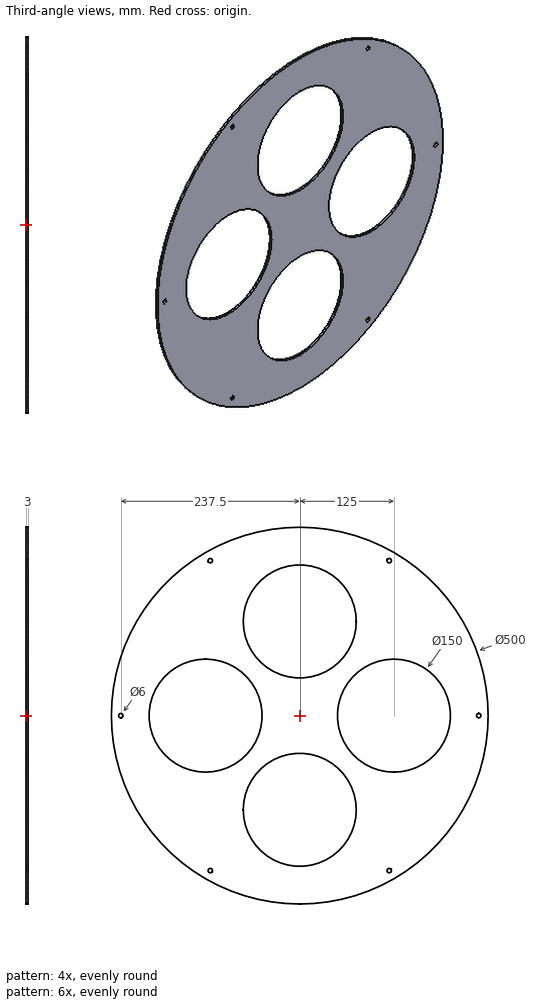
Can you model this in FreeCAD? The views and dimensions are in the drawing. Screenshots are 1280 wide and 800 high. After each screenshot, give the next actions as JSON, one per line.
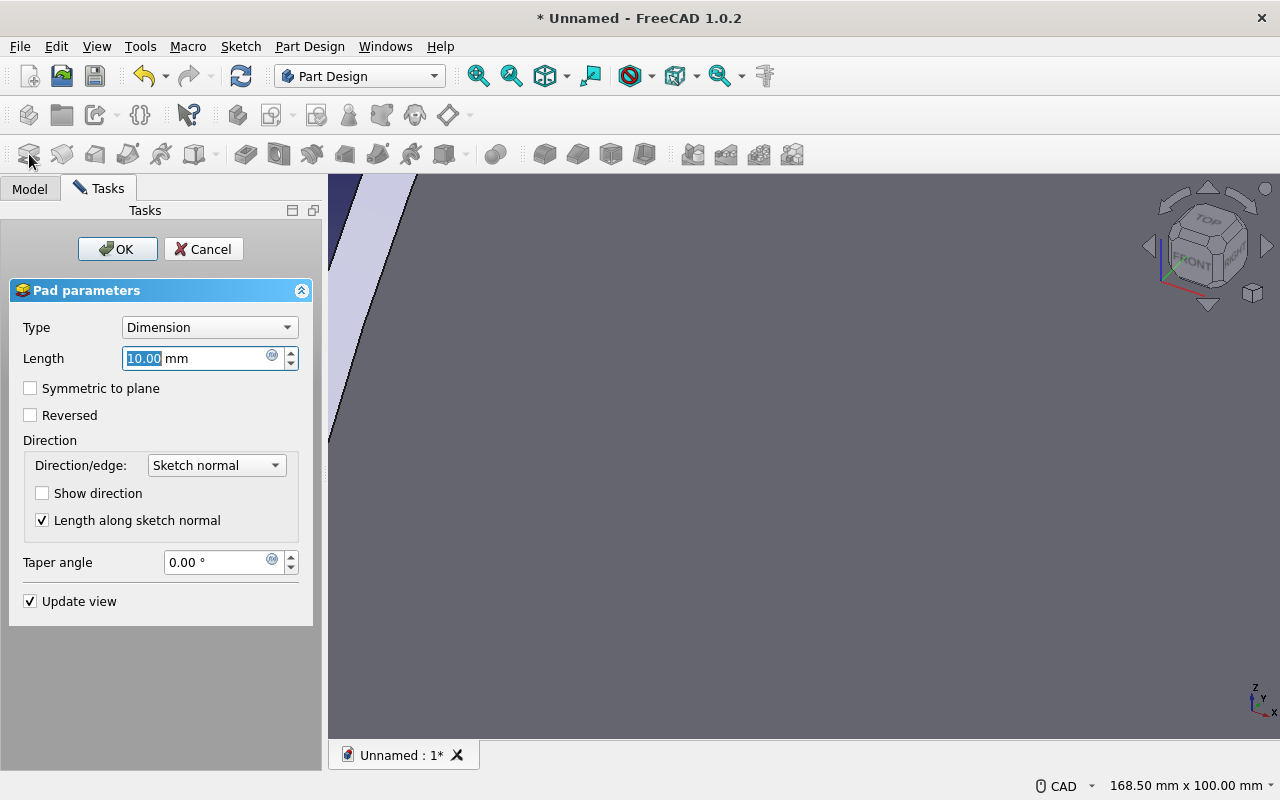
{"action": "type", "text": "3"}
{"action": "key", "text": "Tab"}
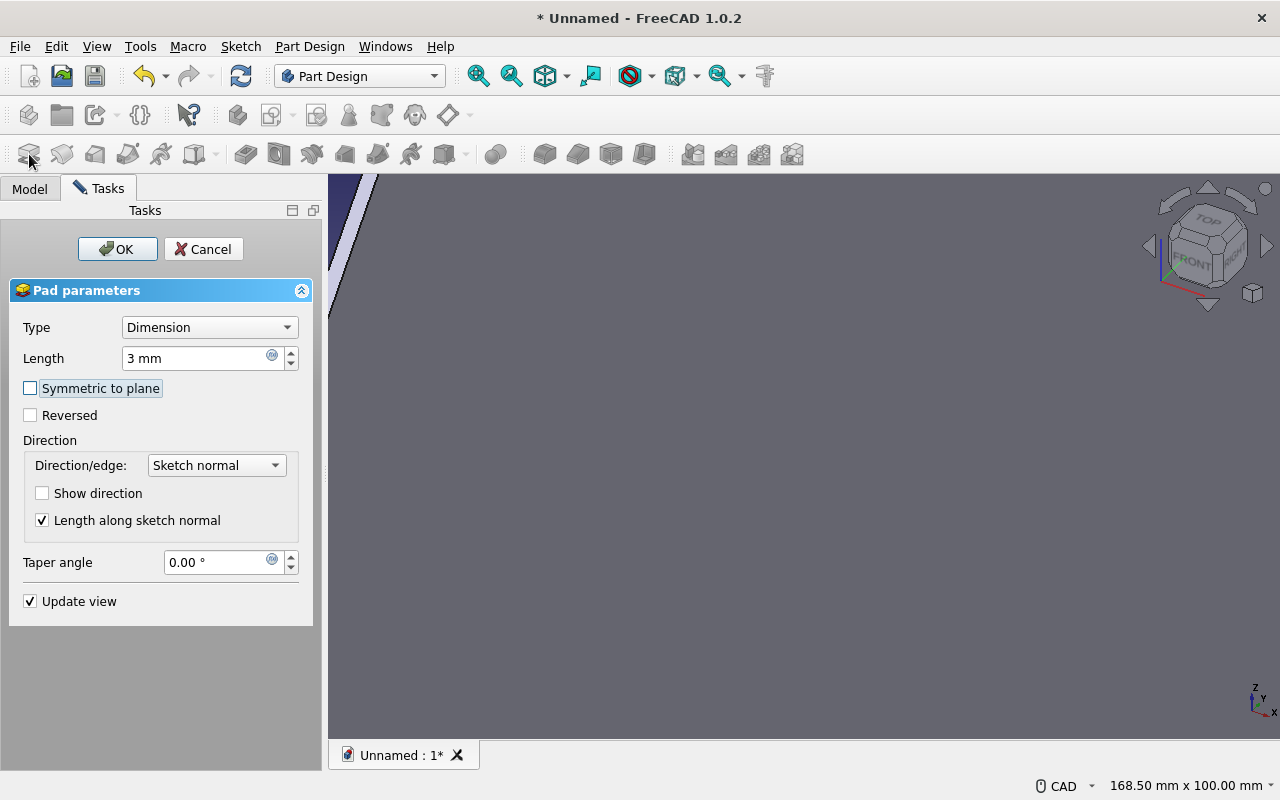
{"action": "left_click", "coordinate": [118, 249]}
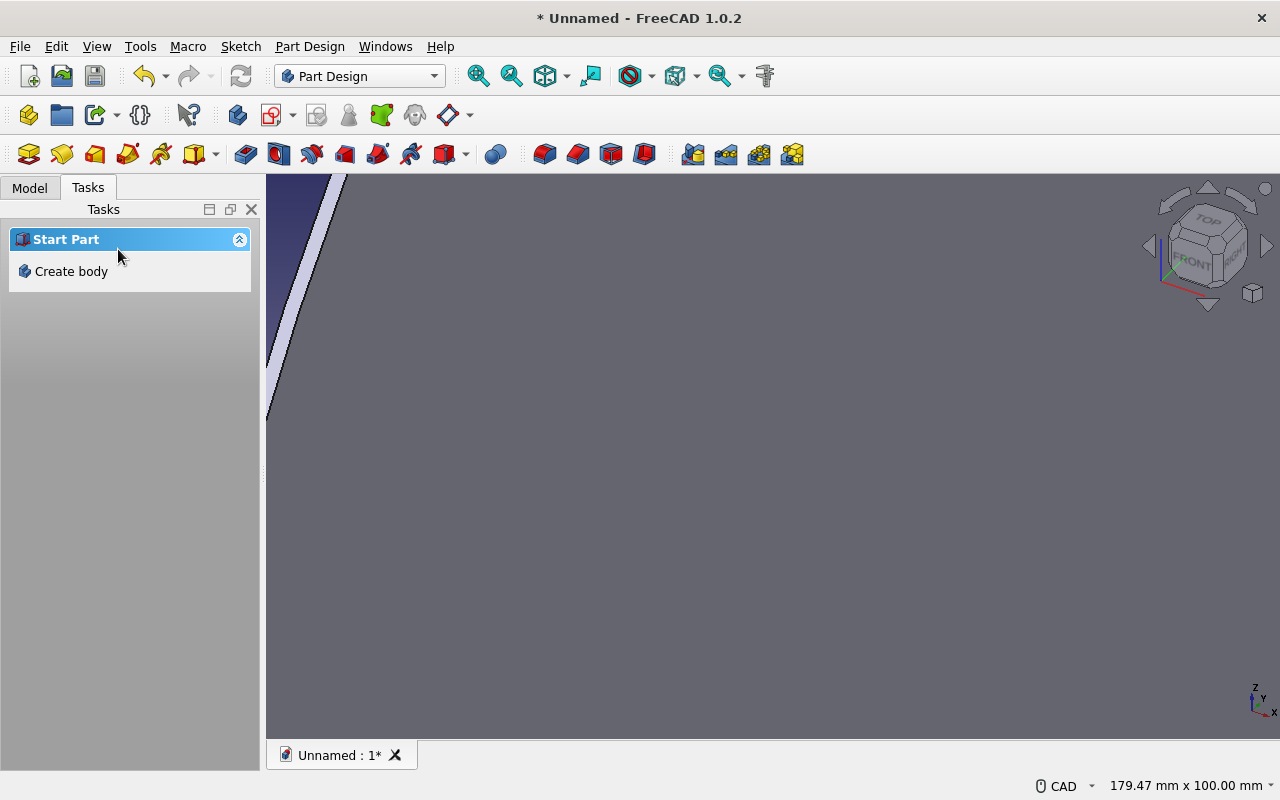
{"action": "left_click", "coordinate": [479, 76]}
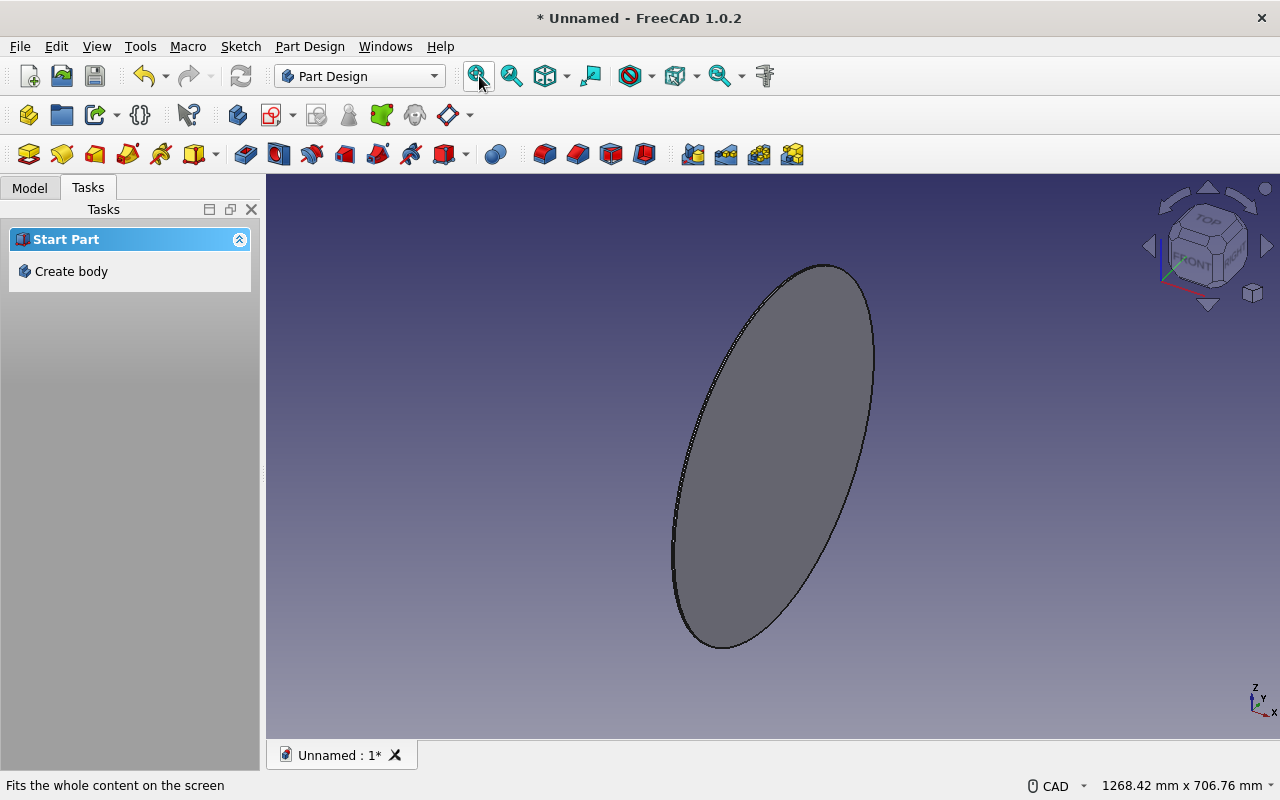
{"action": "left_click", "coordinate": [774, 456]}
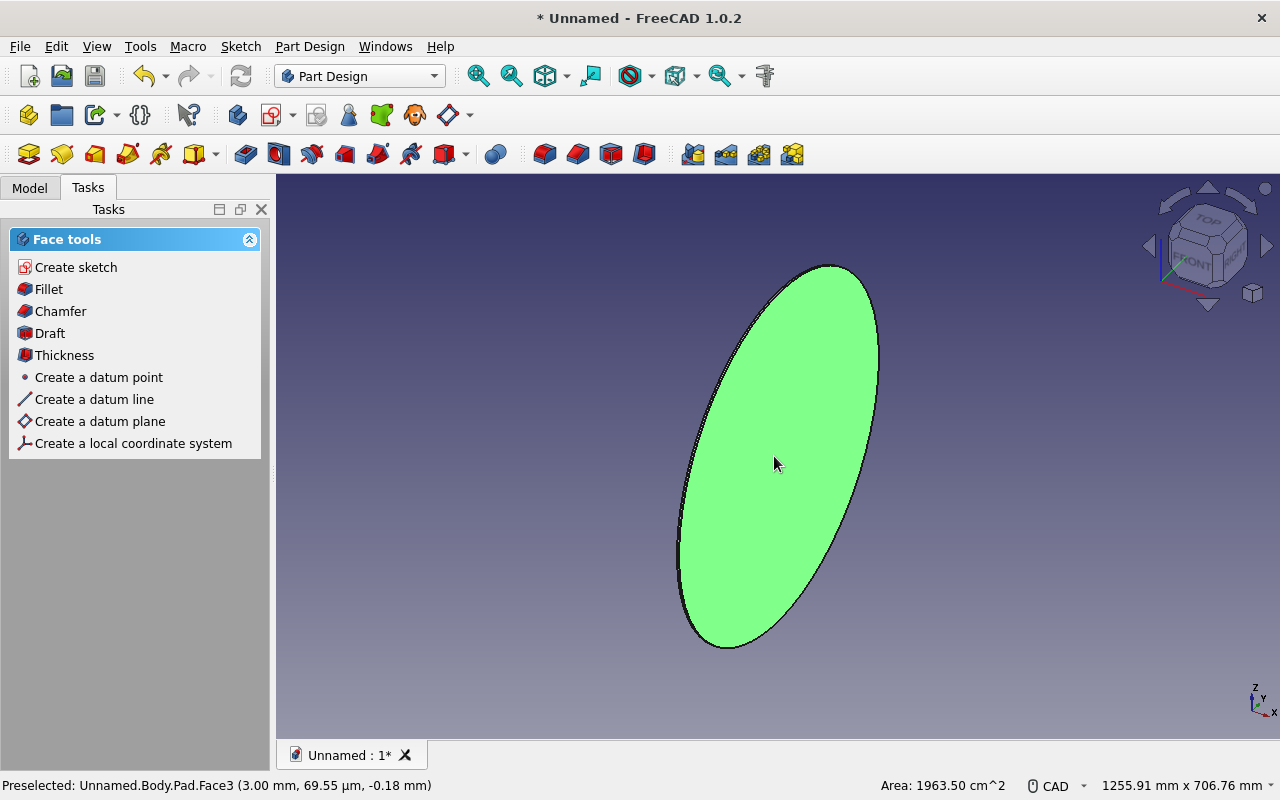
{"action": "left_click", "coordinate": [270, 116]}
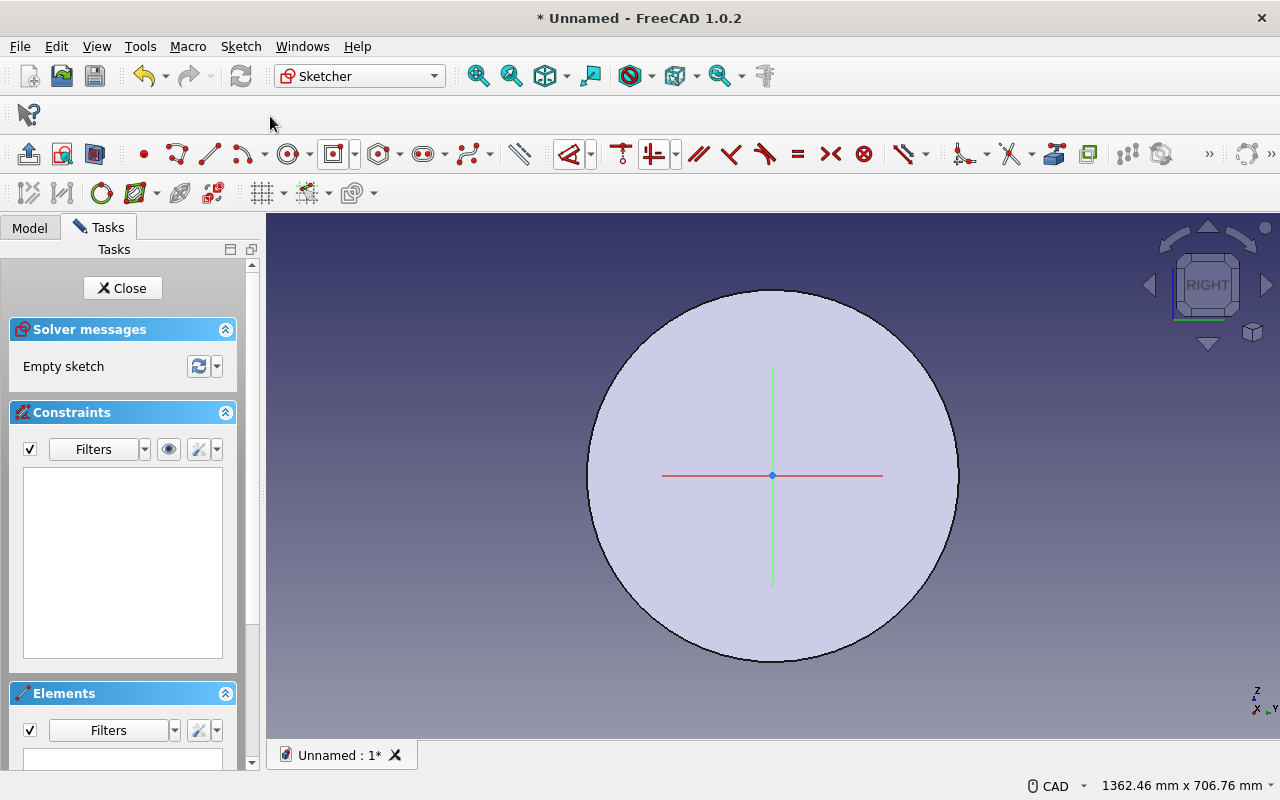
{"action": "scroll", "coordinate": [930, 476], "scroll_direction": "up", "scroll_amount": 5}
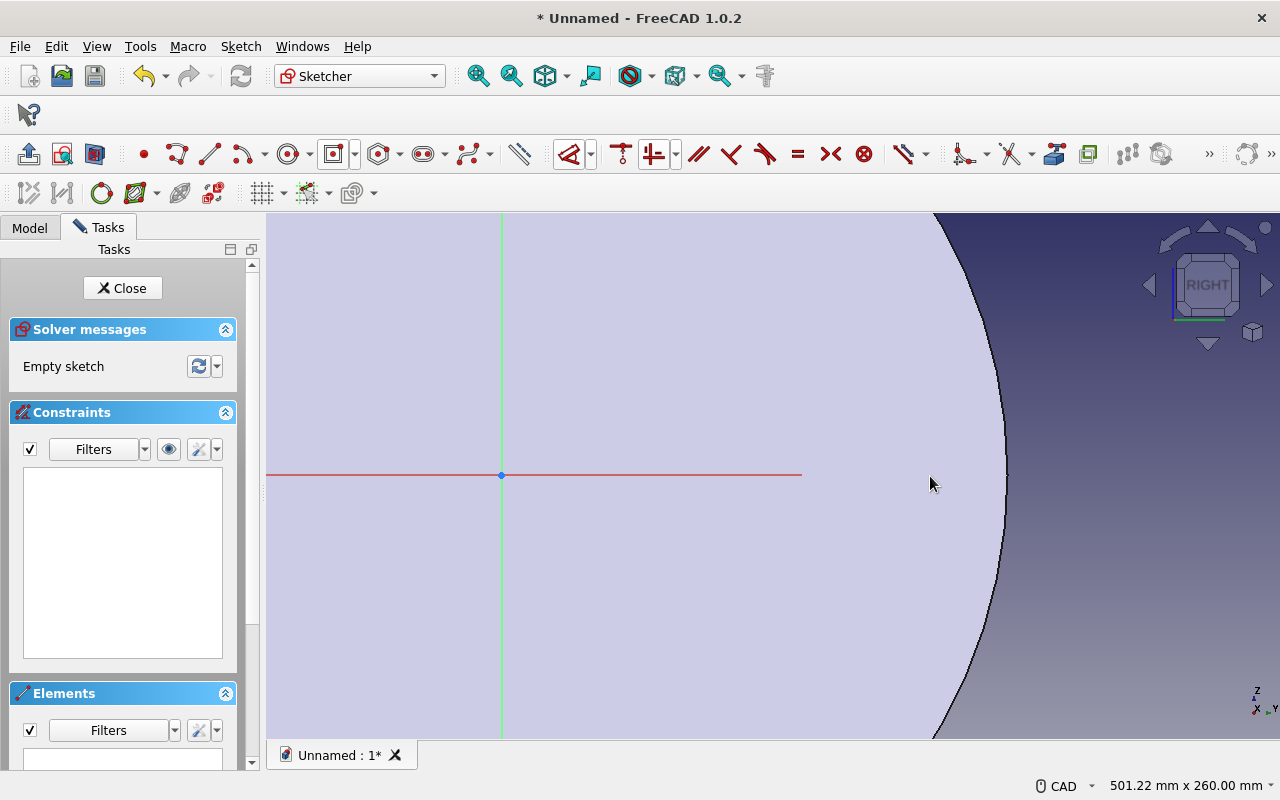
{"action": "left_click", "coordinate": [288, 154]}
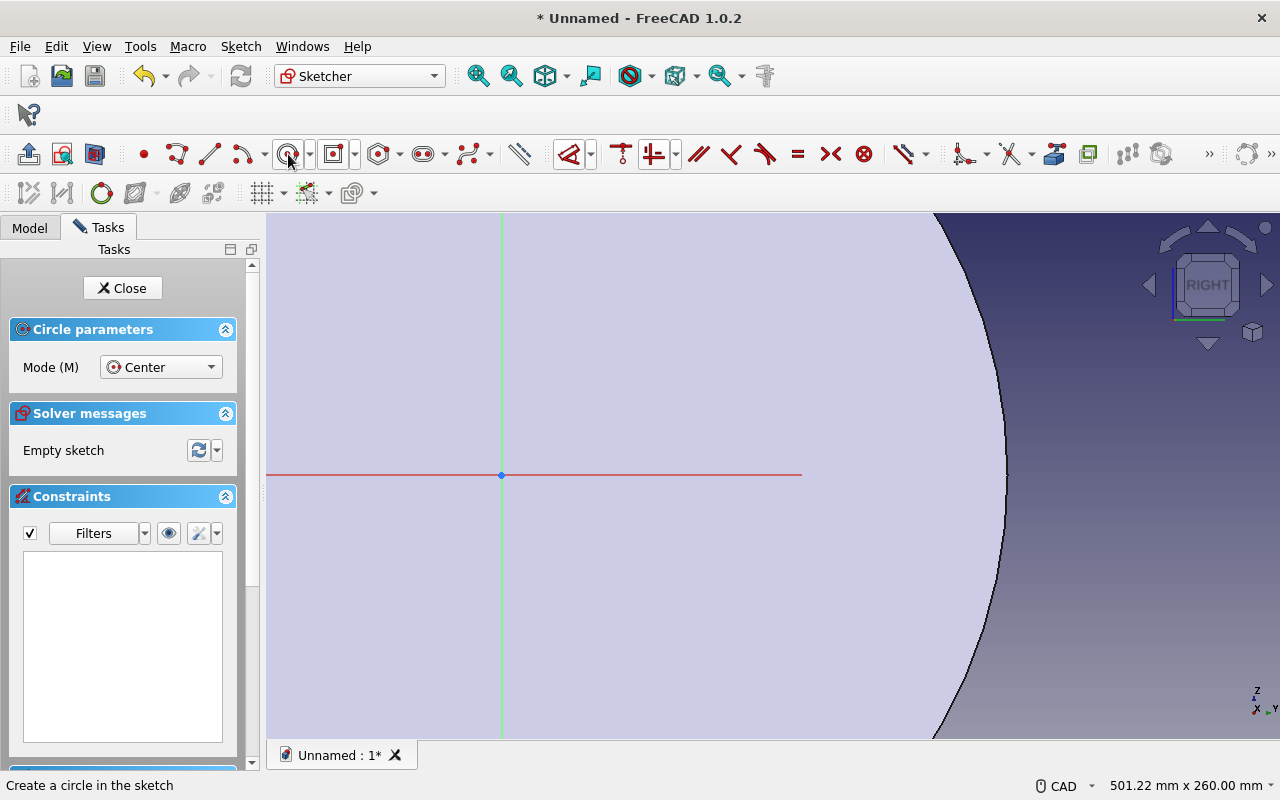
{"action": "left_click", "coordinate": [755, 475]}
{"action": "mouse_move", "coordinate": [862, 368]}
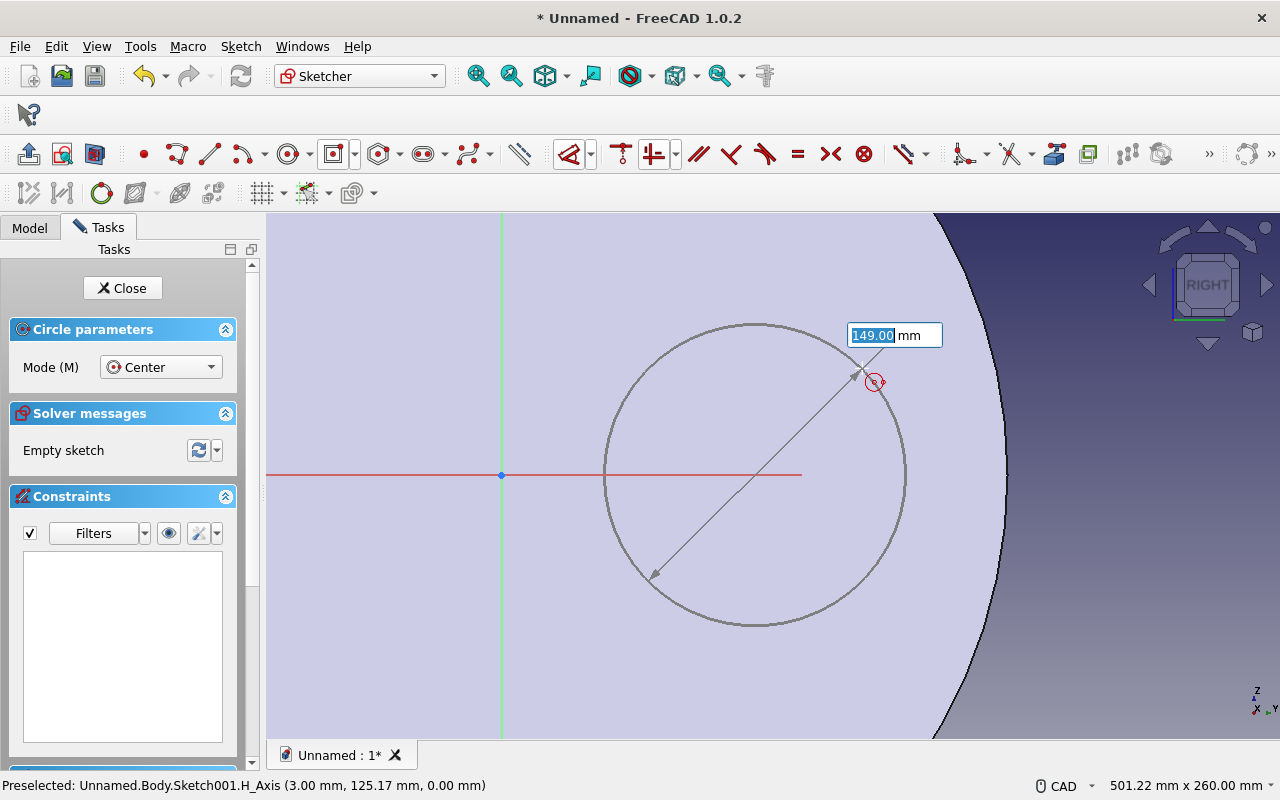
{"action": "type", "text": "150"}
{"action": "key", "text": "Return"}
{"action": "key", "text": "Escape"}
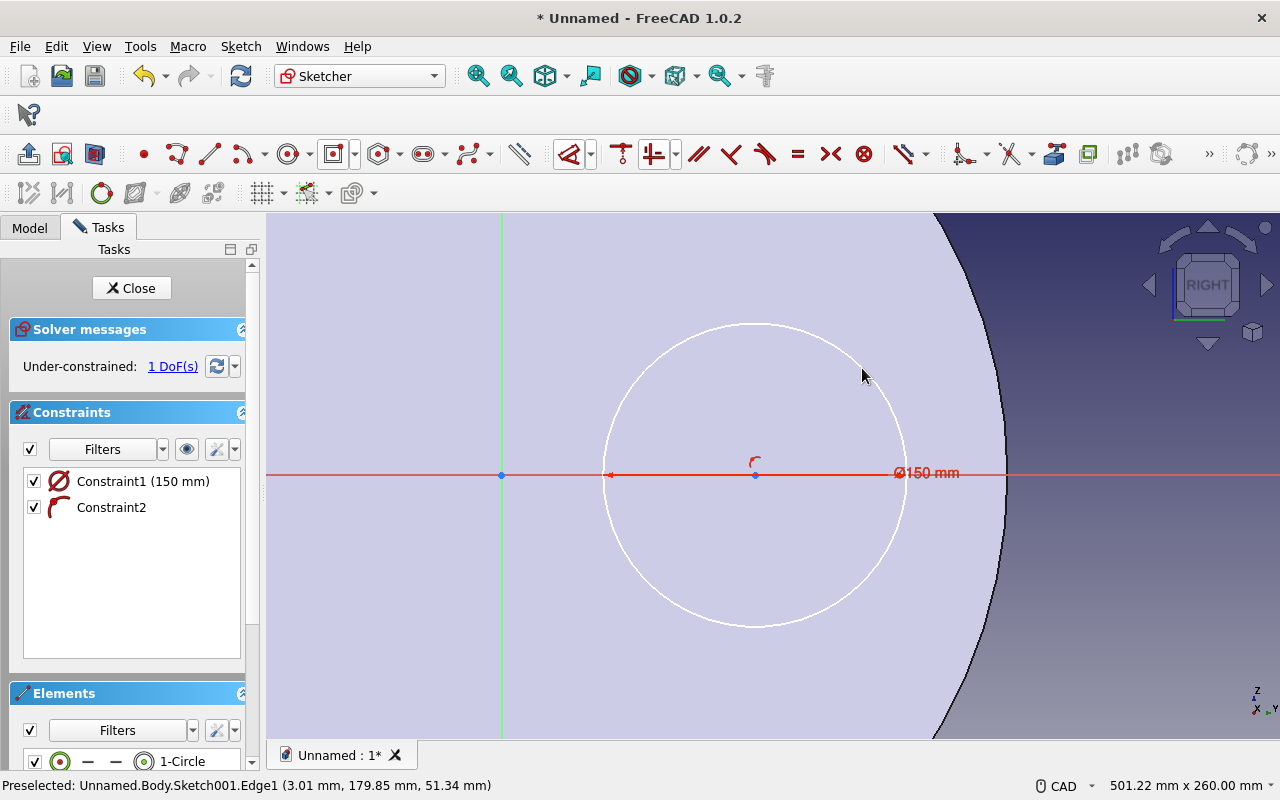
{"action": "left_click", "coordinate": [568, 154]}